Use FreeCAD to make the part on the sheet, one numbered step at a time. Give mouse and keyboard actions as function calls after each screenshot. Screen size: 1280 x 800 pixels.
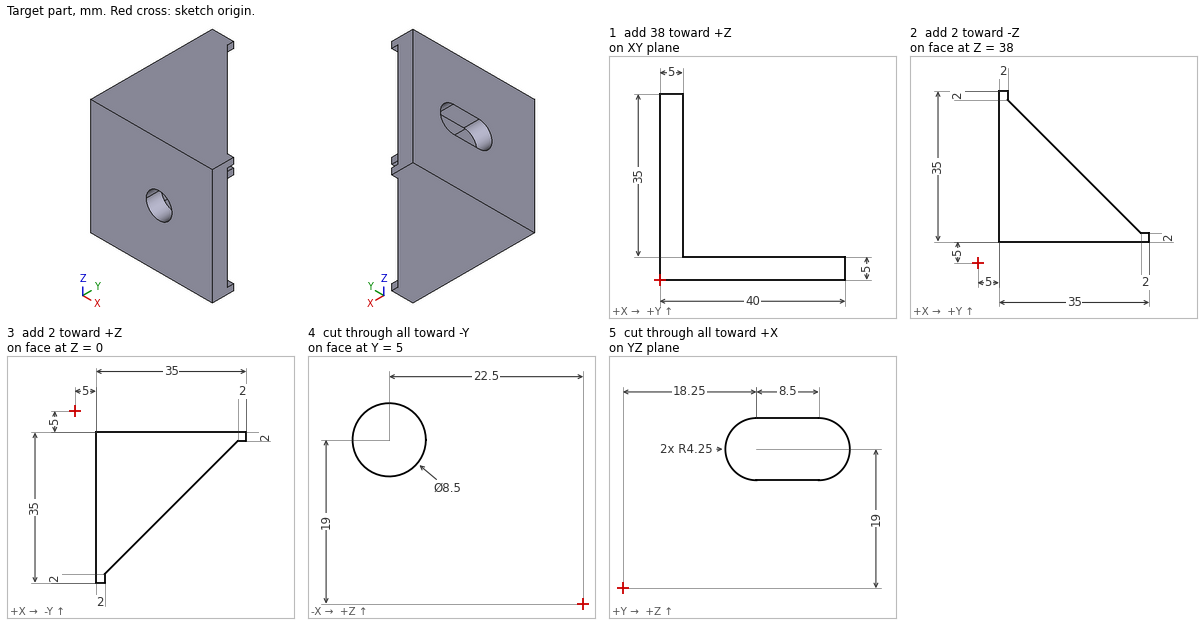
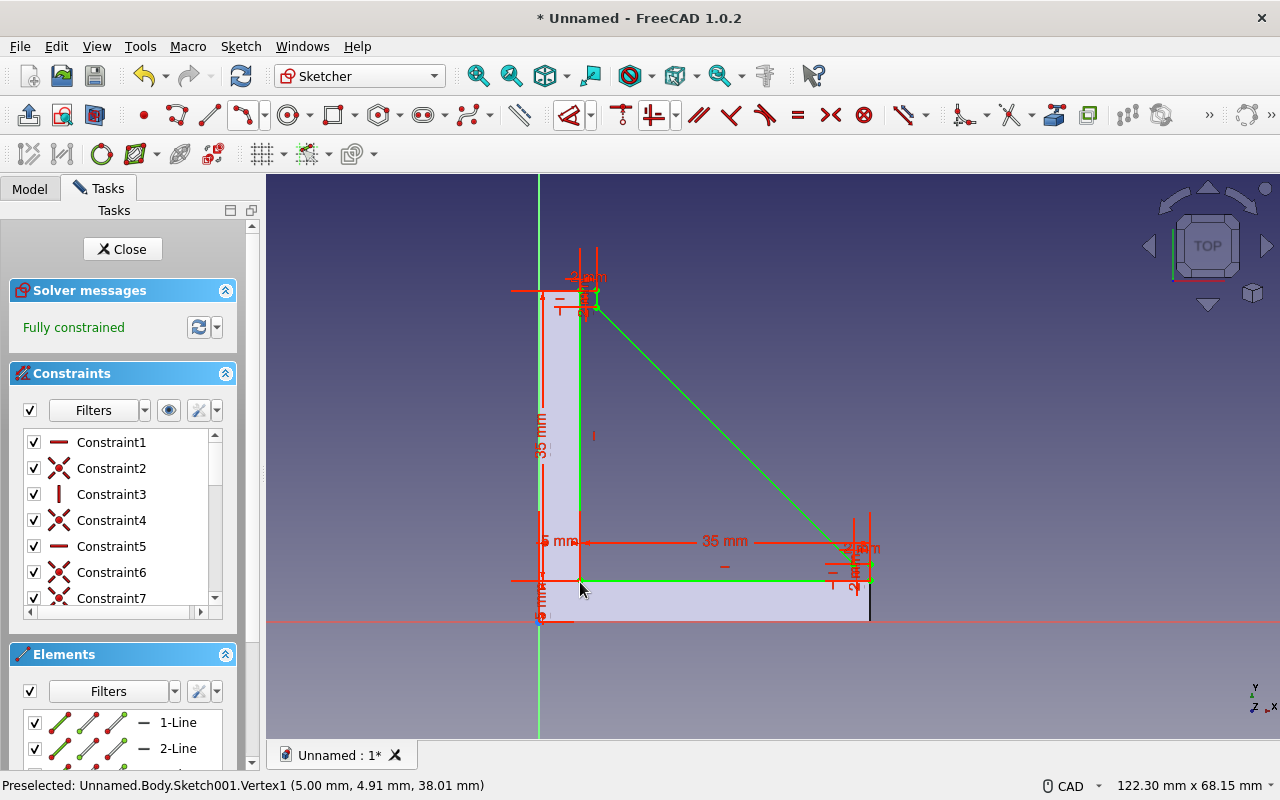
click(123, 249)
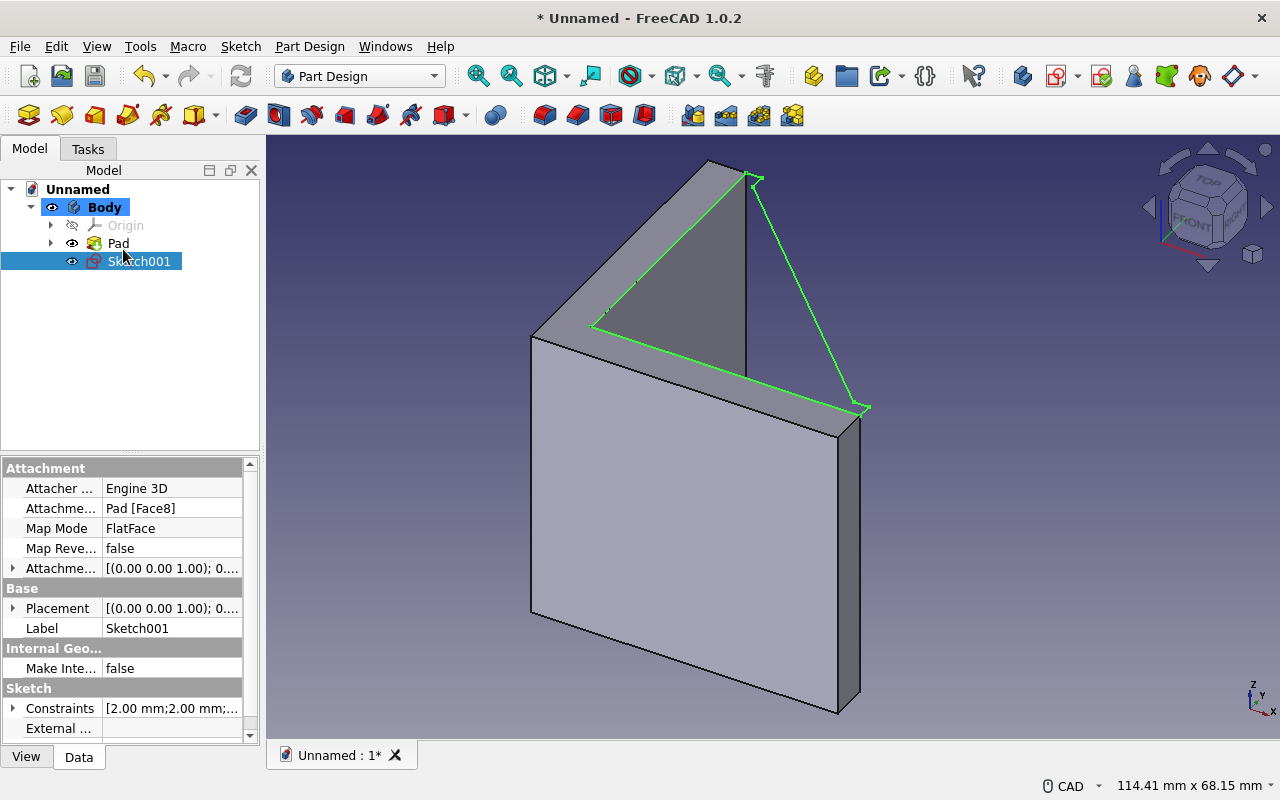
click(29, 116)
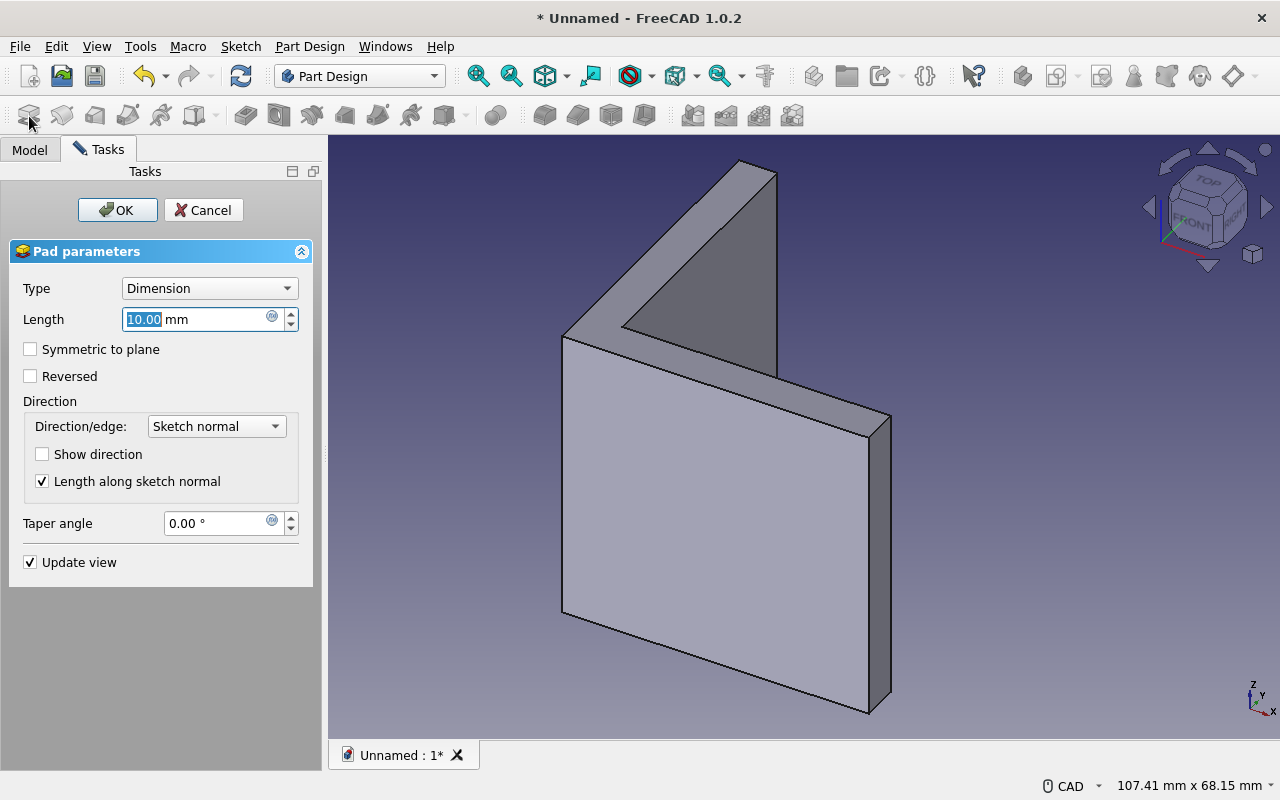
text(2)
key(Tab)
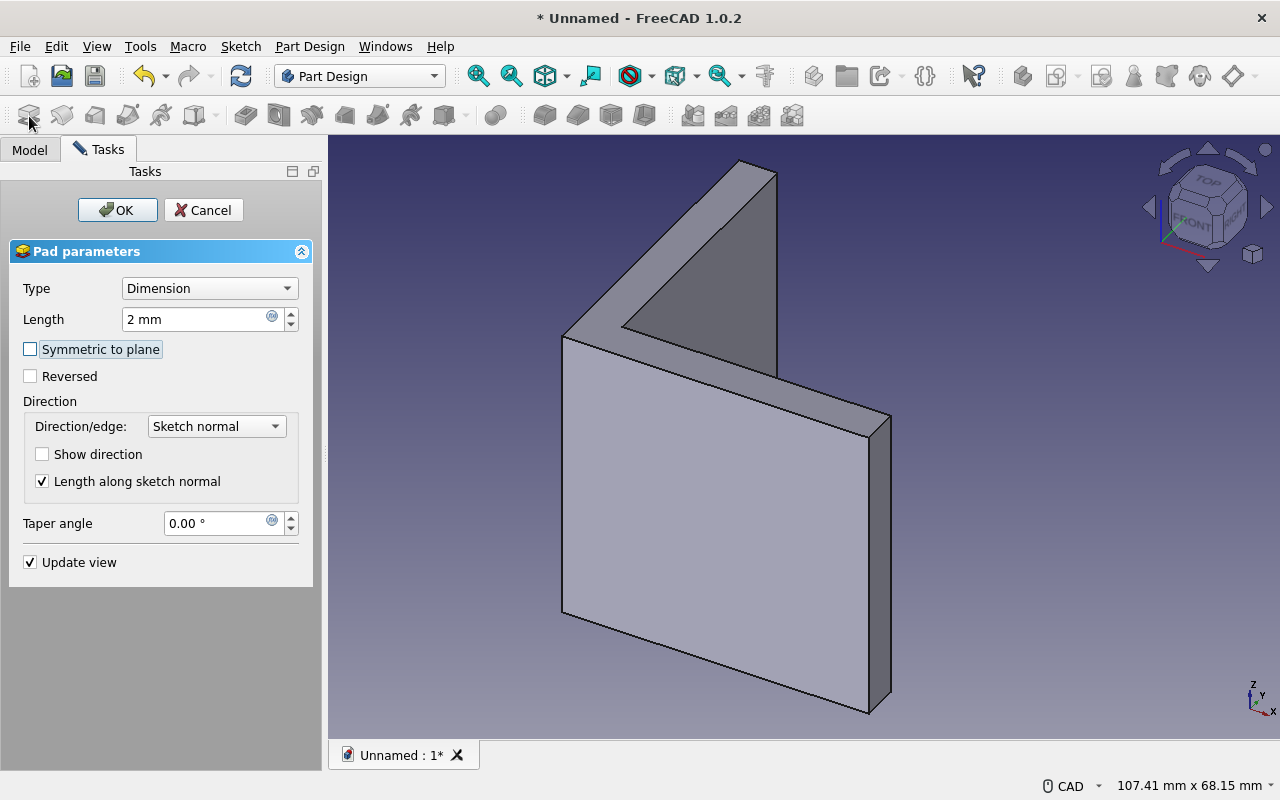
click(31, 376)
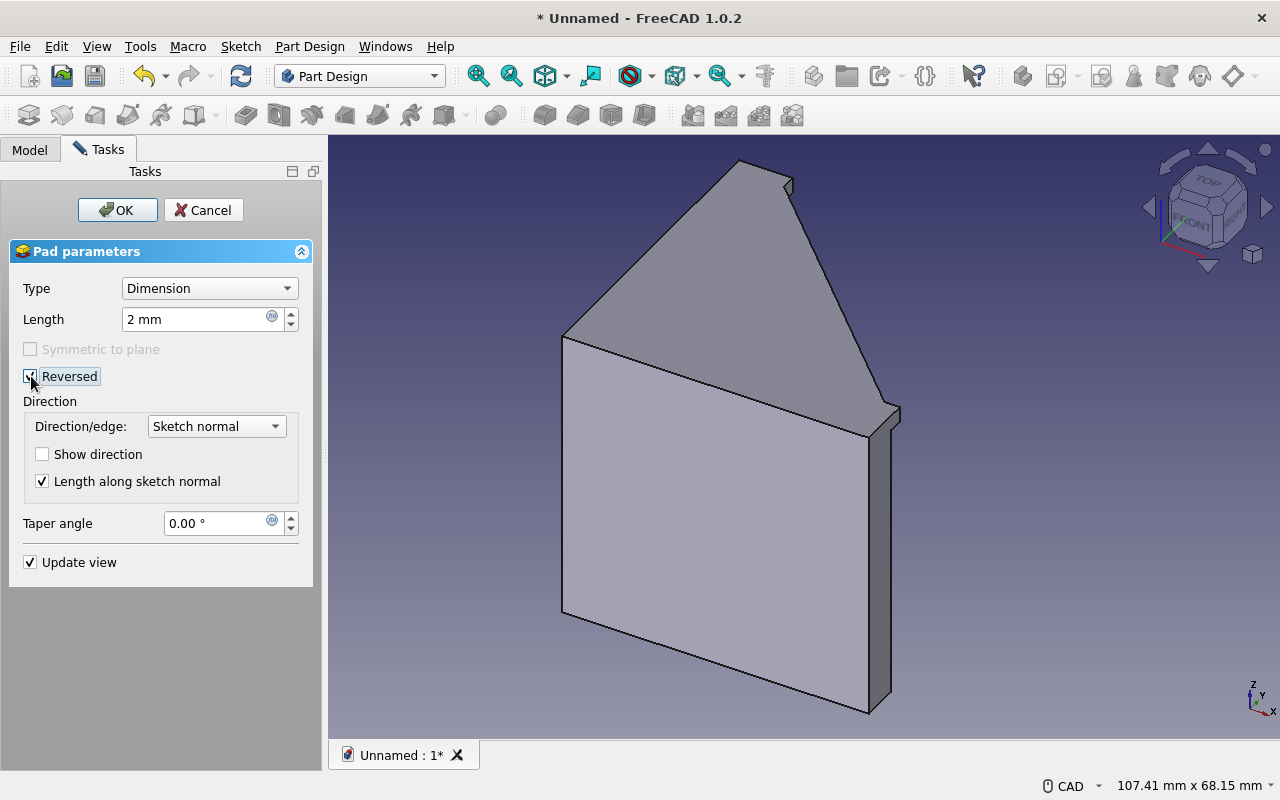
click(118, 210)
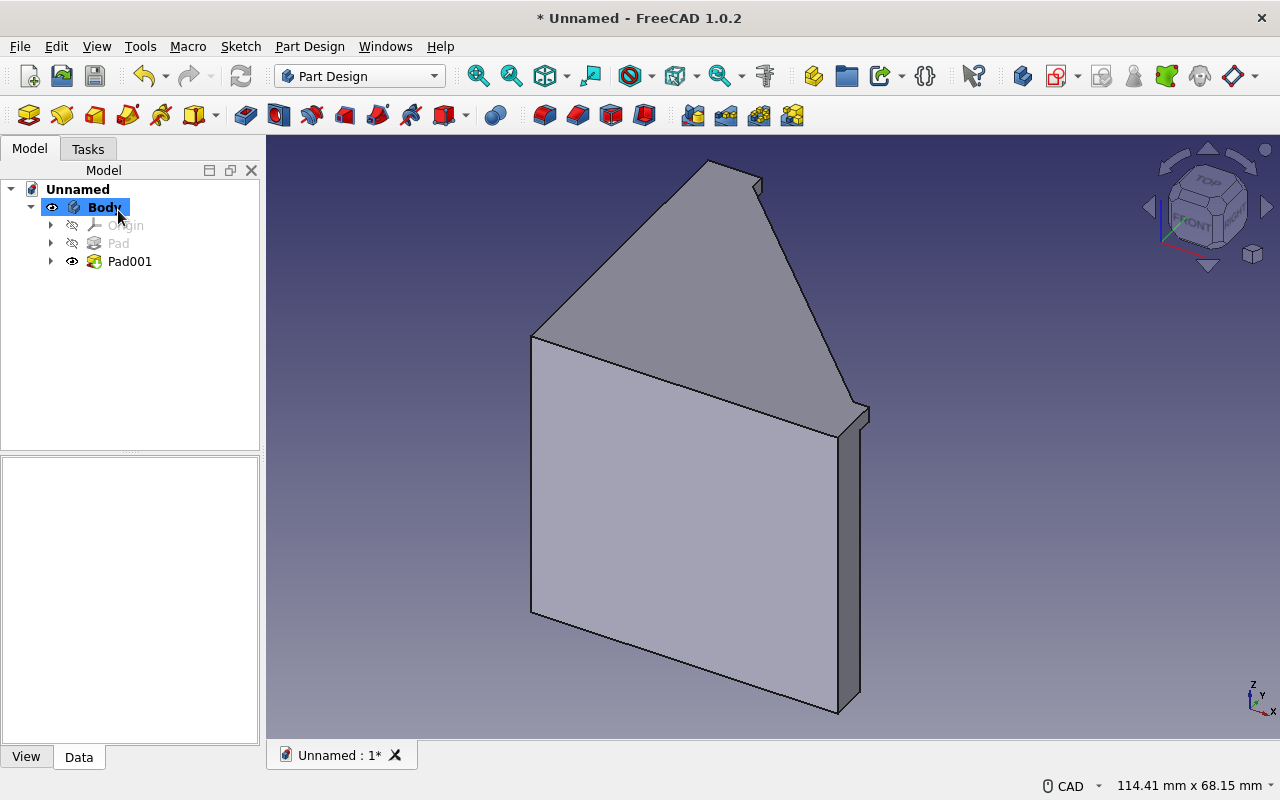
key(5)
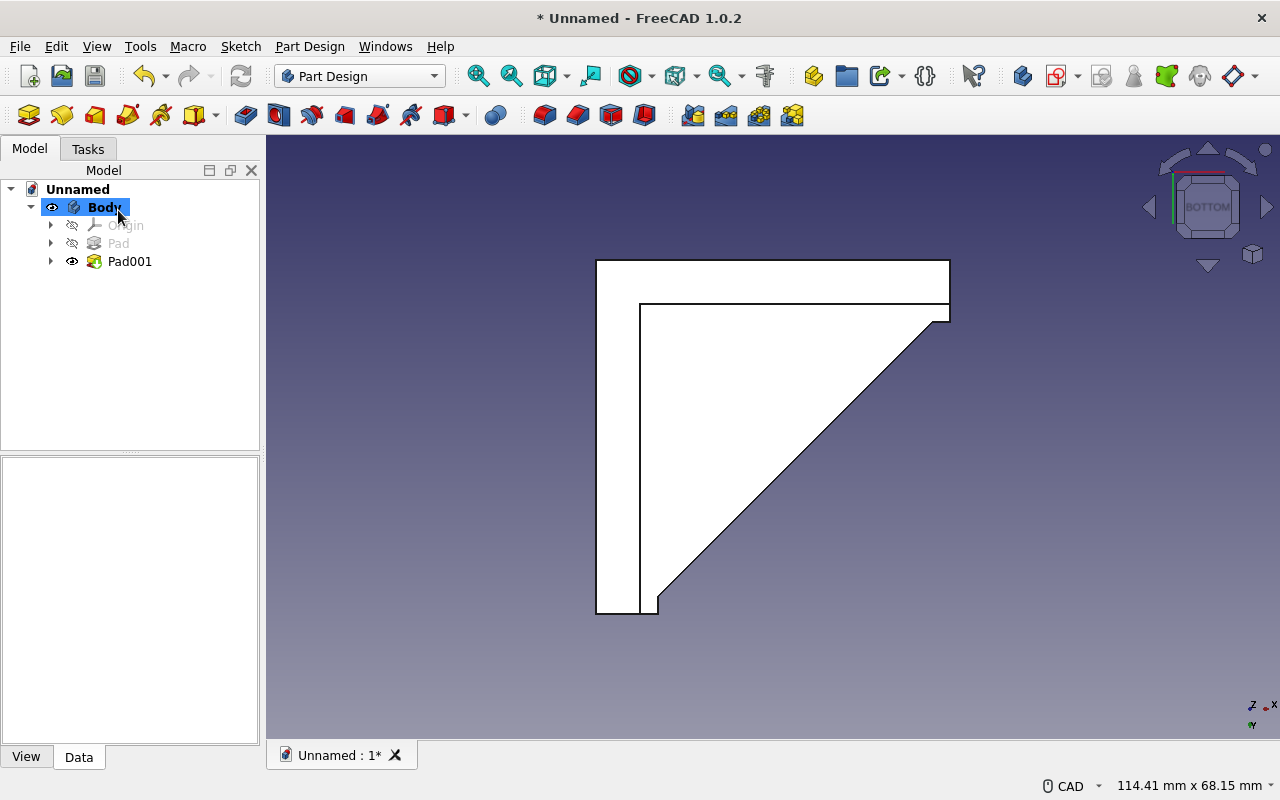
click(621, 284)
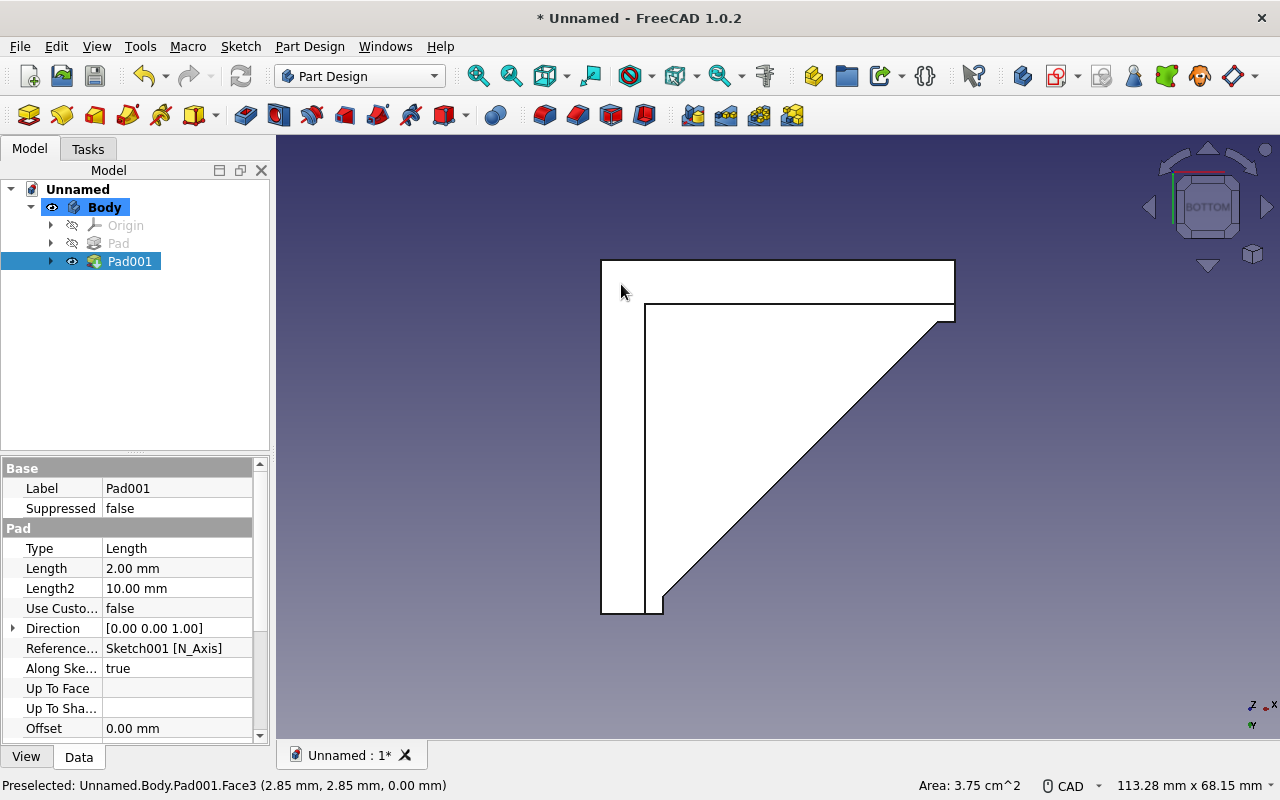
click(1056, 76)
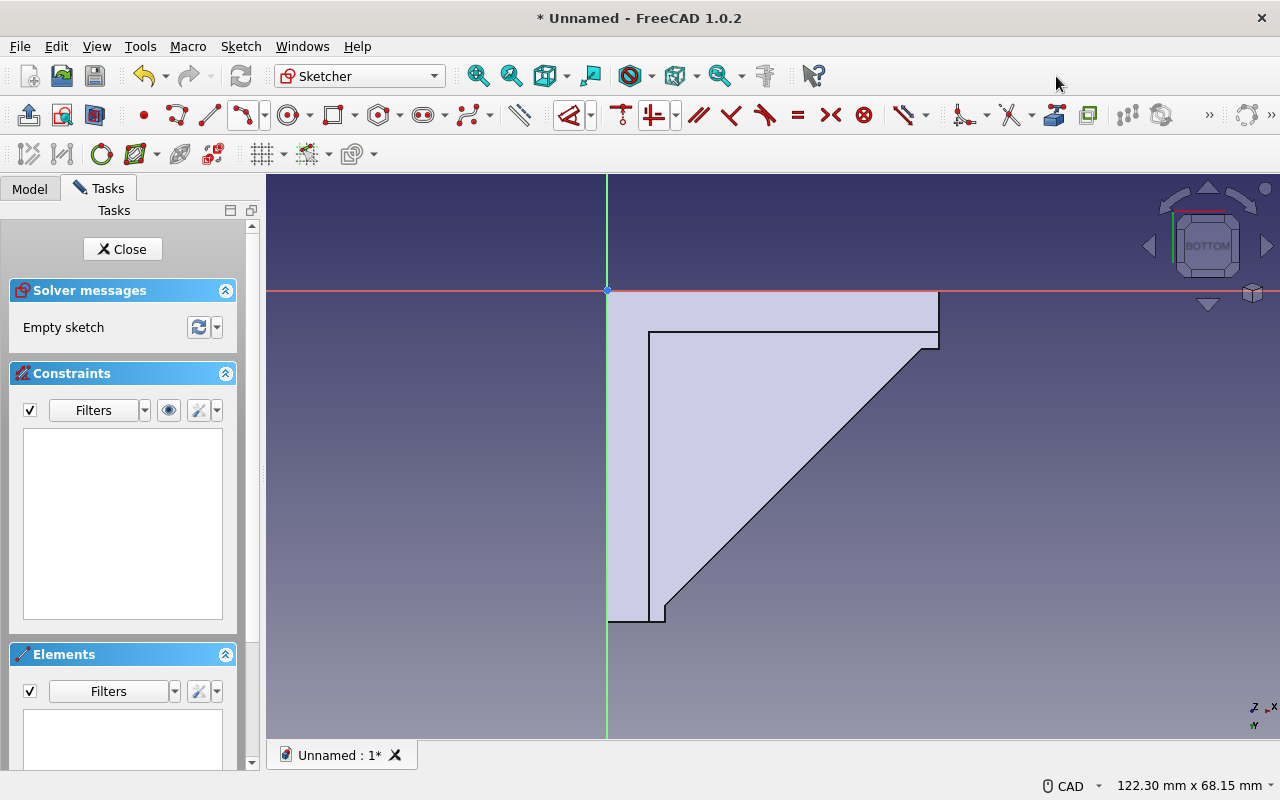
click(177, 116)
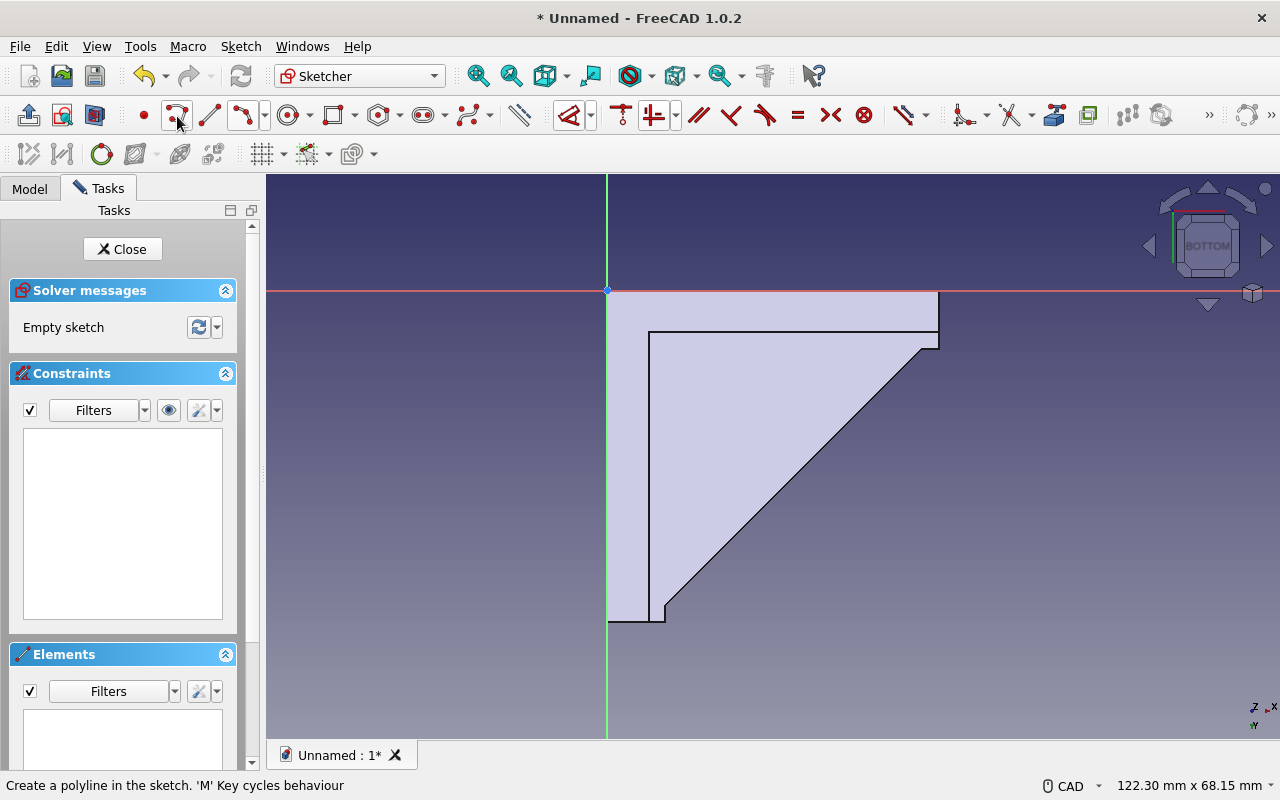
click(649, 332)
click(649, 622)
click(665, 622)
click(665, 606)
click(922, 349)
click(939, 349)
click(939, 332)
click(649, 333)
key(Escape)
key(Escape)